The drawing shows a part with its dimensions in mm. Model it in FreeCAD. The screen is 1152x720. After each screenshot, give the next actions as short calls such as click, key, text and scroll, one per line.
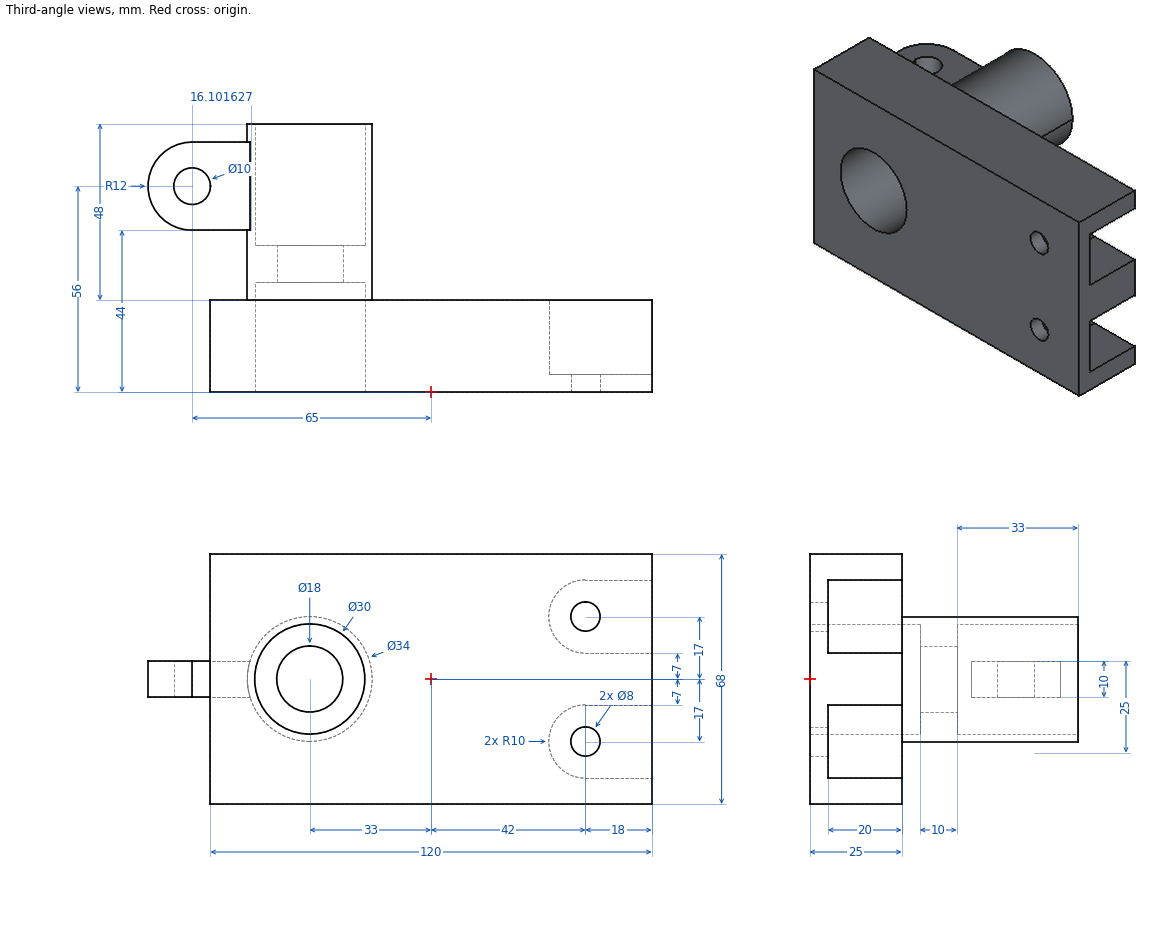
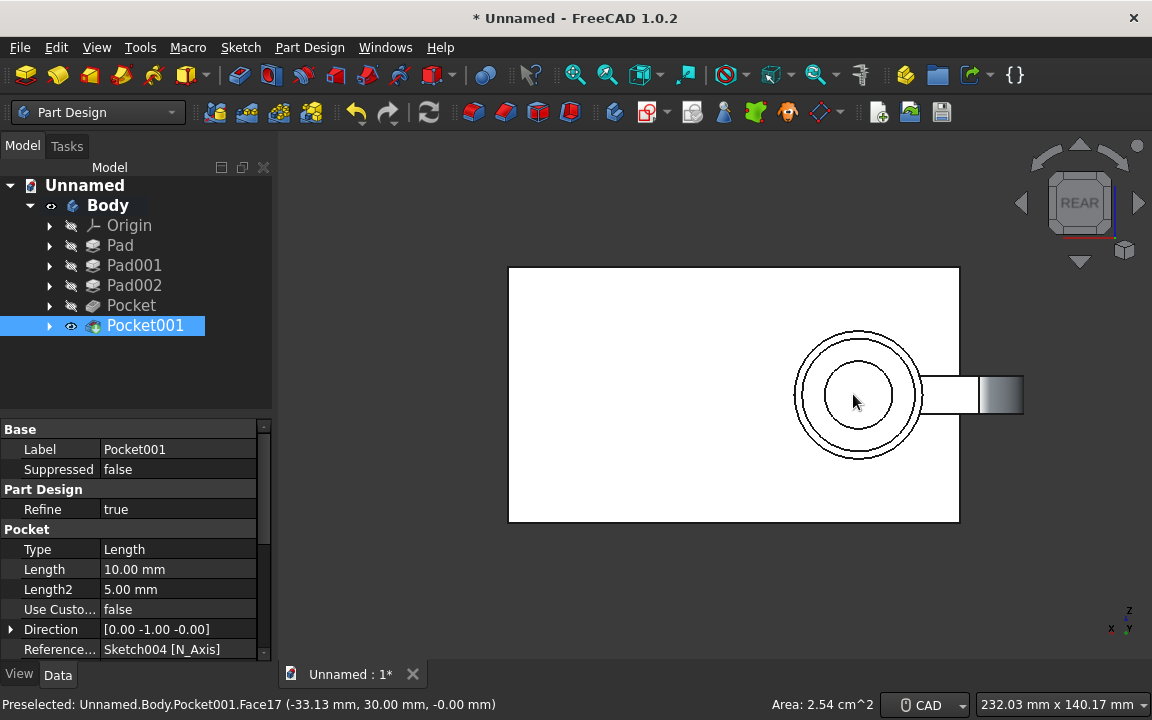
click(648, 112)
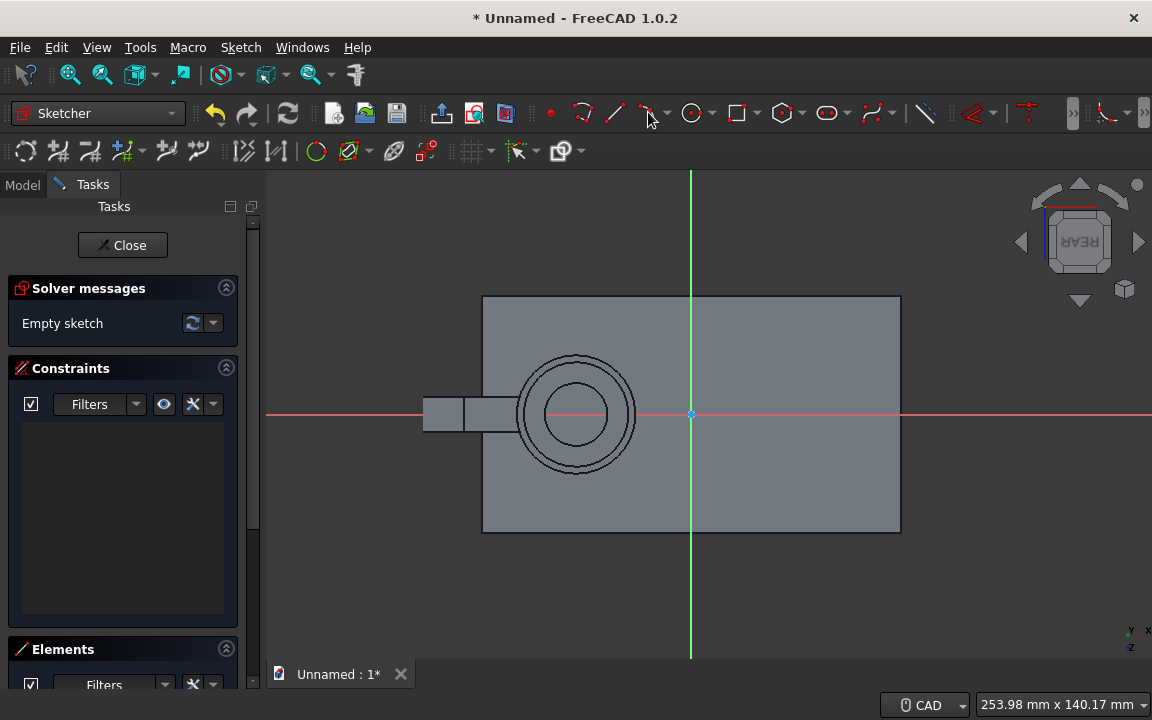
scroll(588, 414, up, 5)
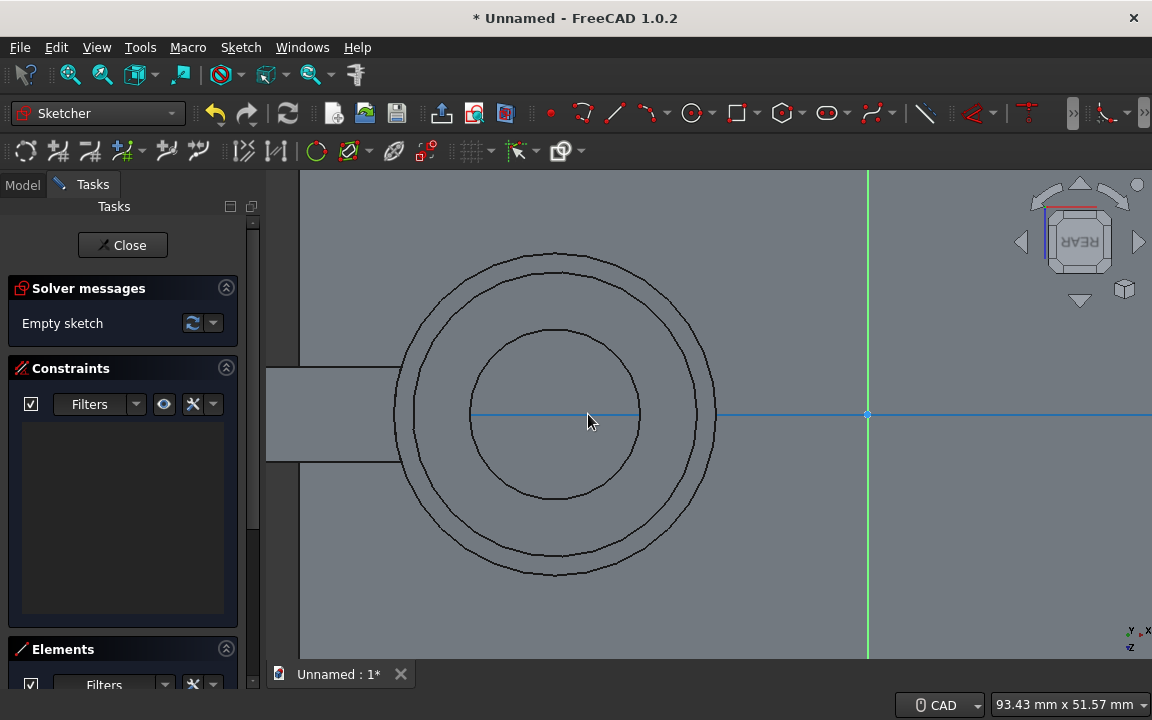
click(692, 114)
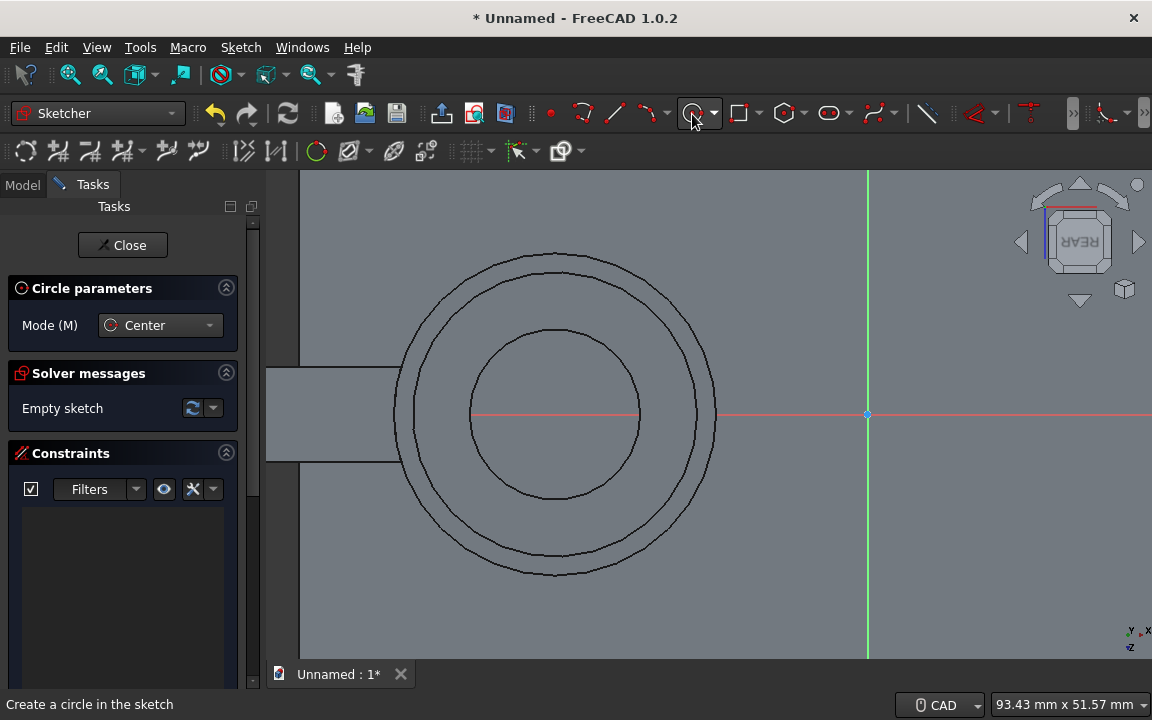
click(555, 414)
move(656, 314)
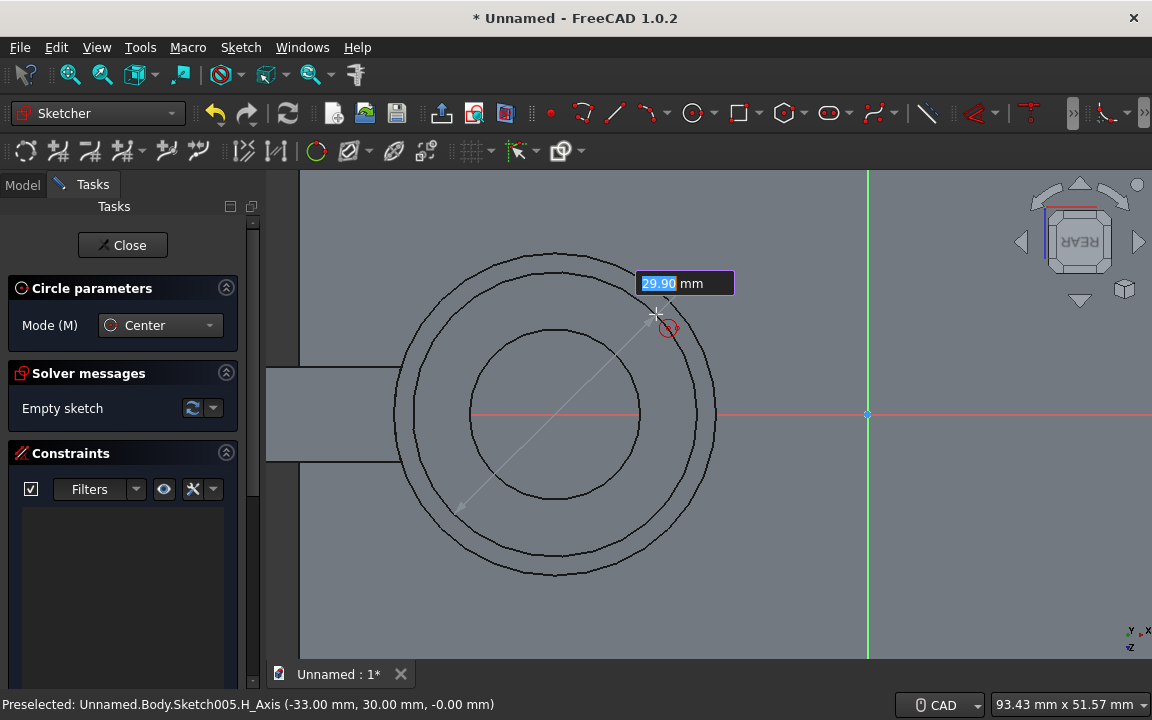
text(30)
key(Return)
key(Escape)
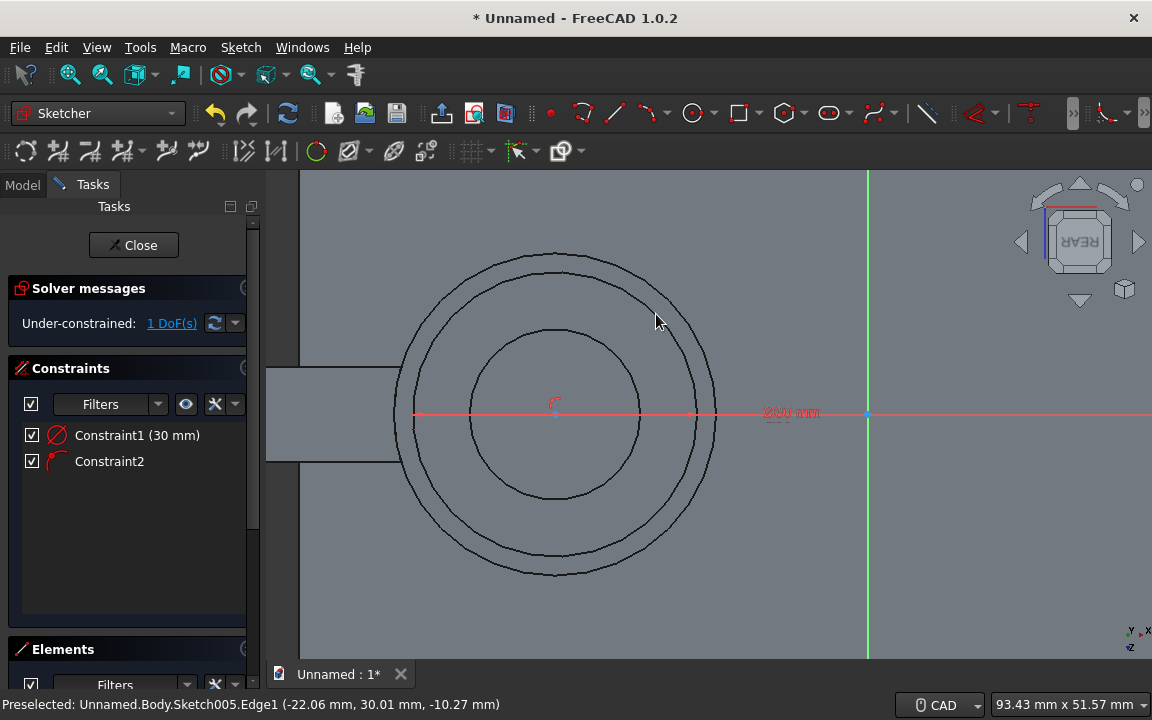
click(974, 114)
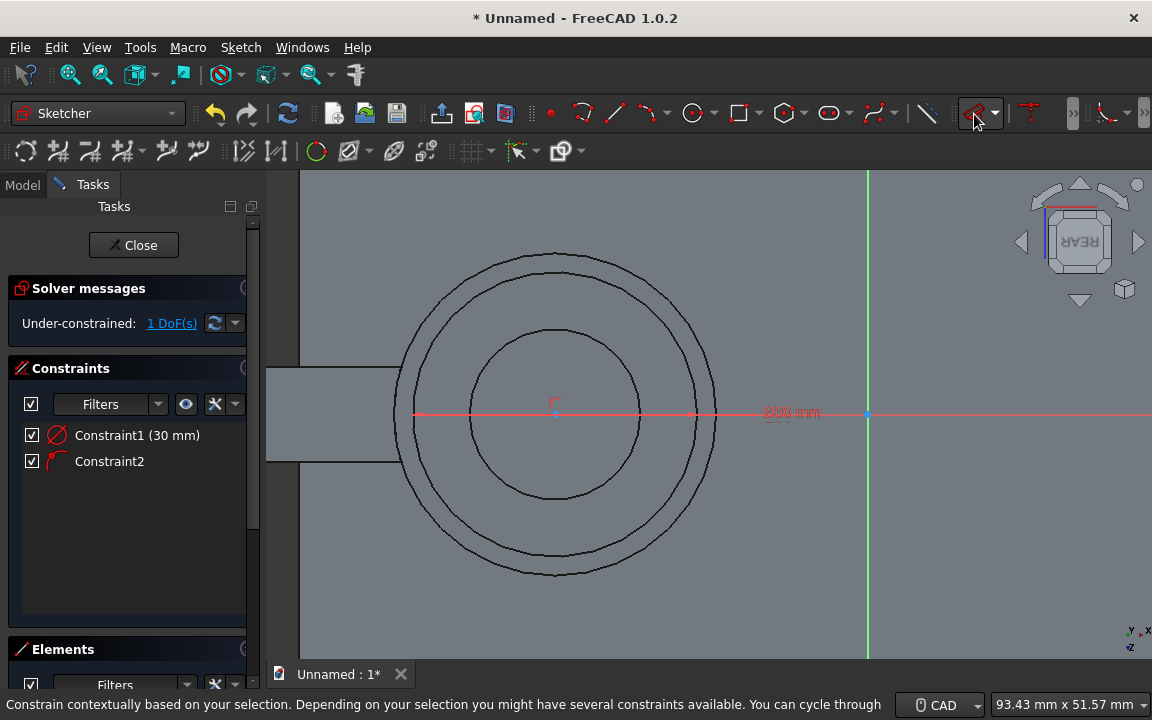
click(555, 414)
click(711, 448)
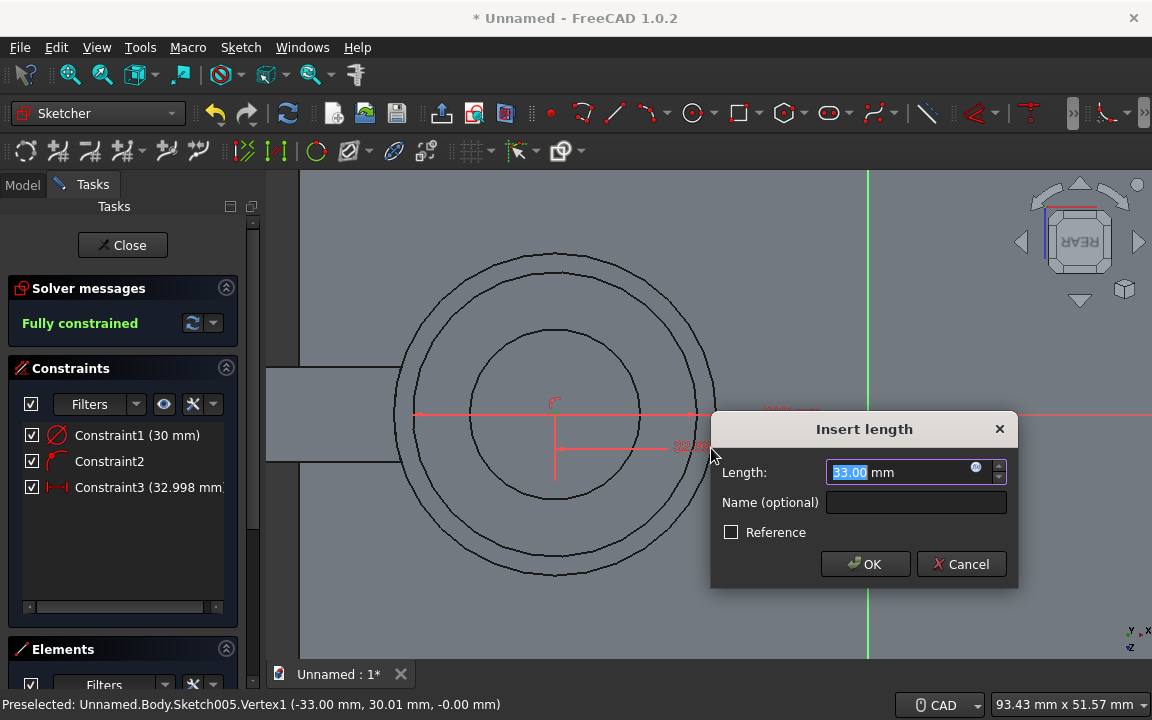
text(33)
key(Return)
key(Escape)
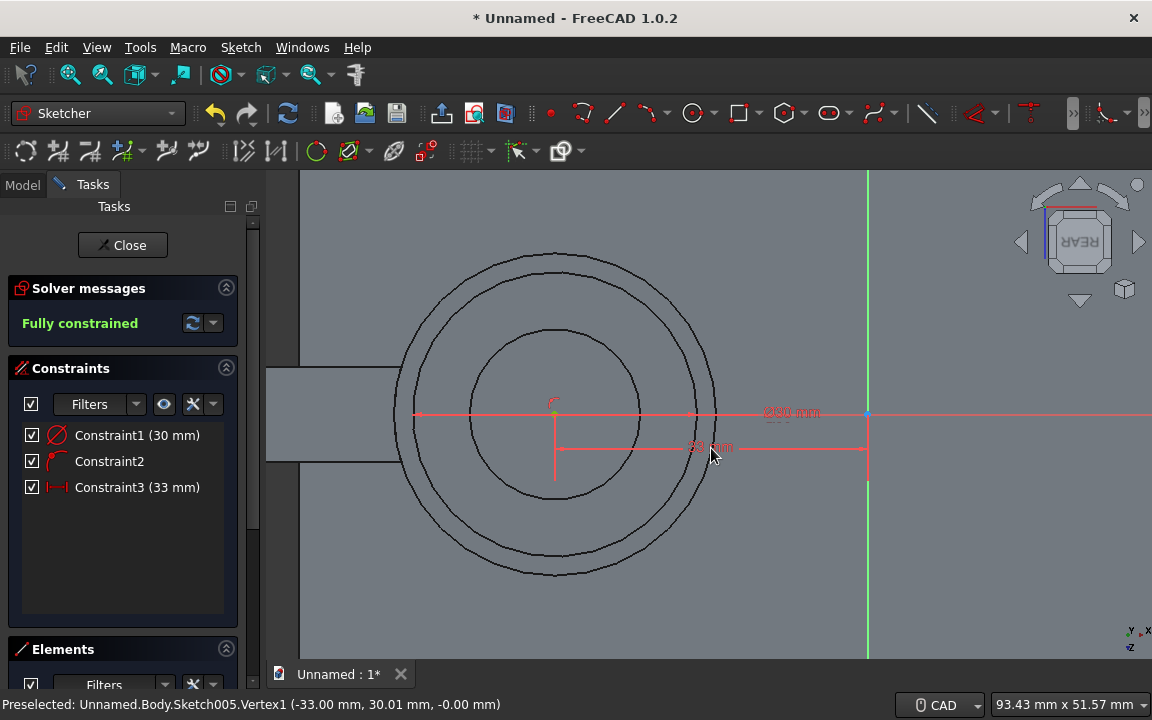
click(123, 245)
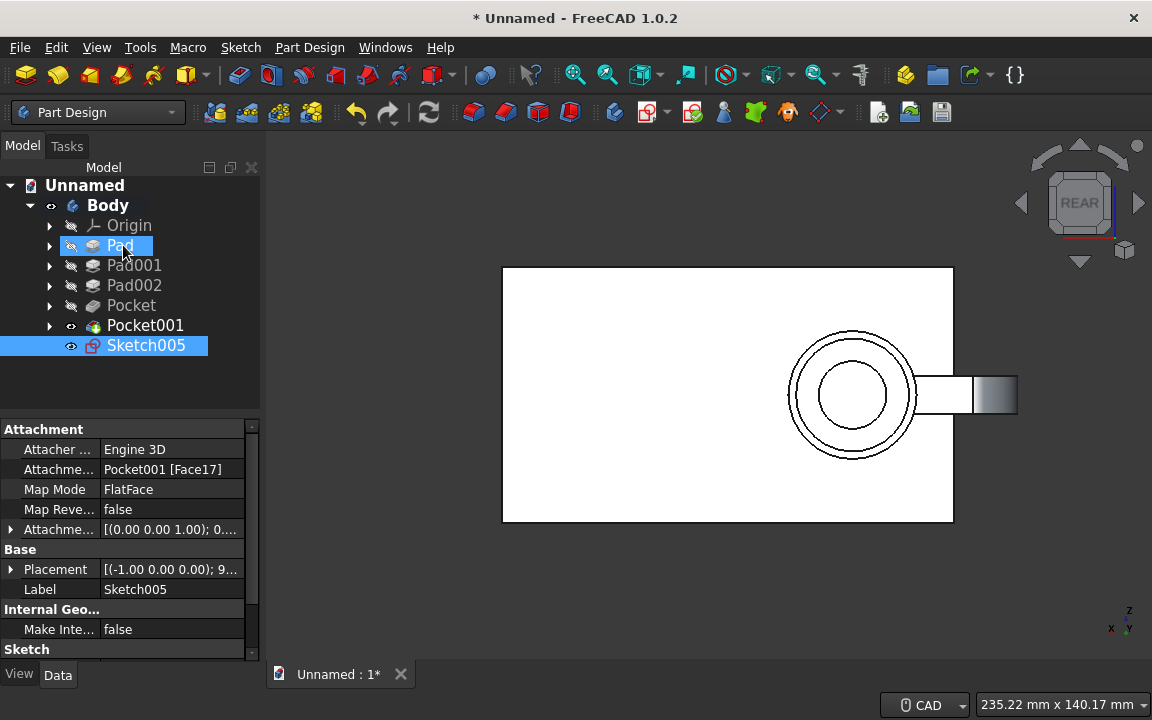
click(240, 76)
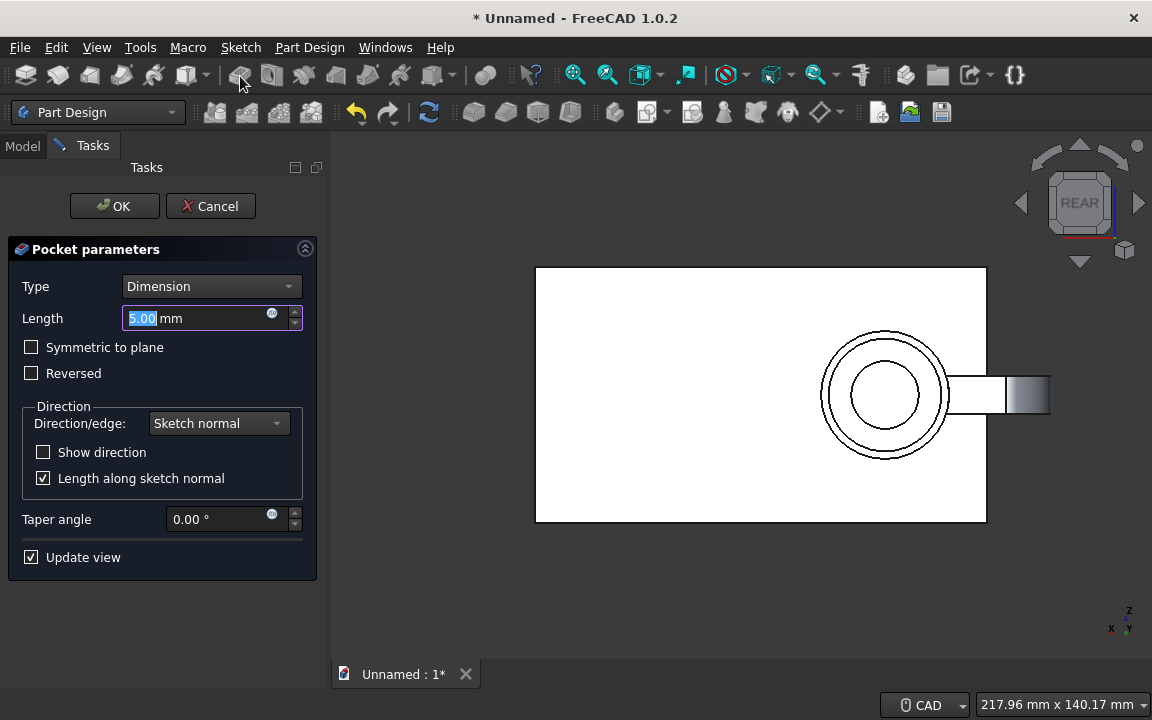
click(212, 286)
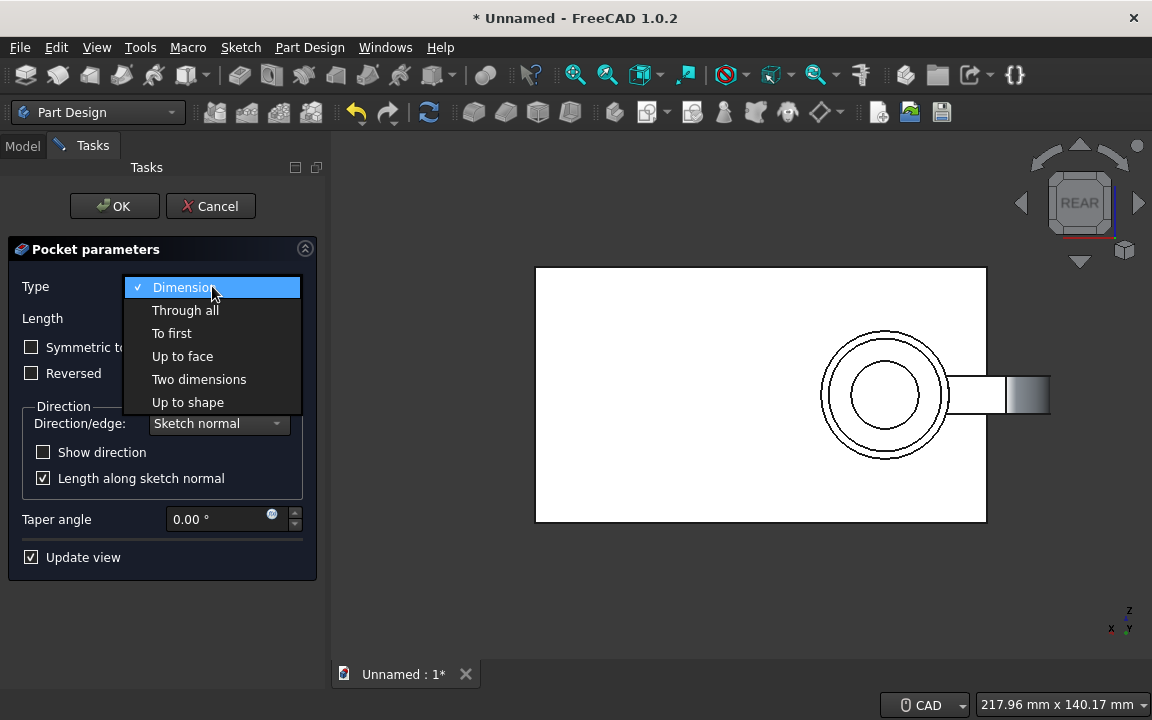
click(212, 310)